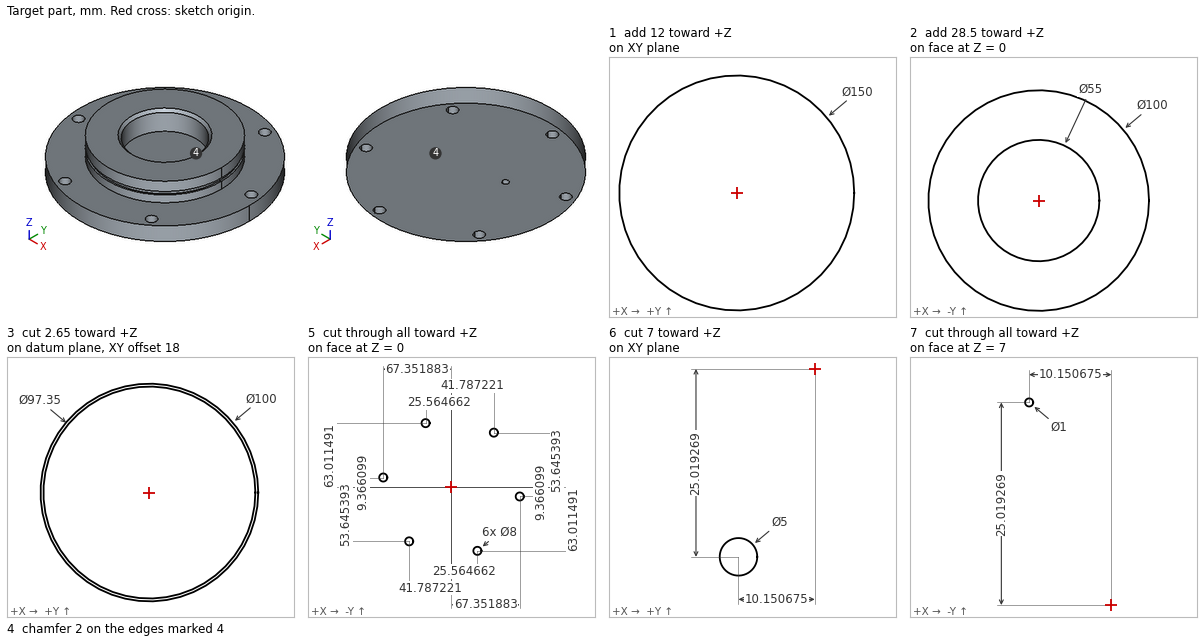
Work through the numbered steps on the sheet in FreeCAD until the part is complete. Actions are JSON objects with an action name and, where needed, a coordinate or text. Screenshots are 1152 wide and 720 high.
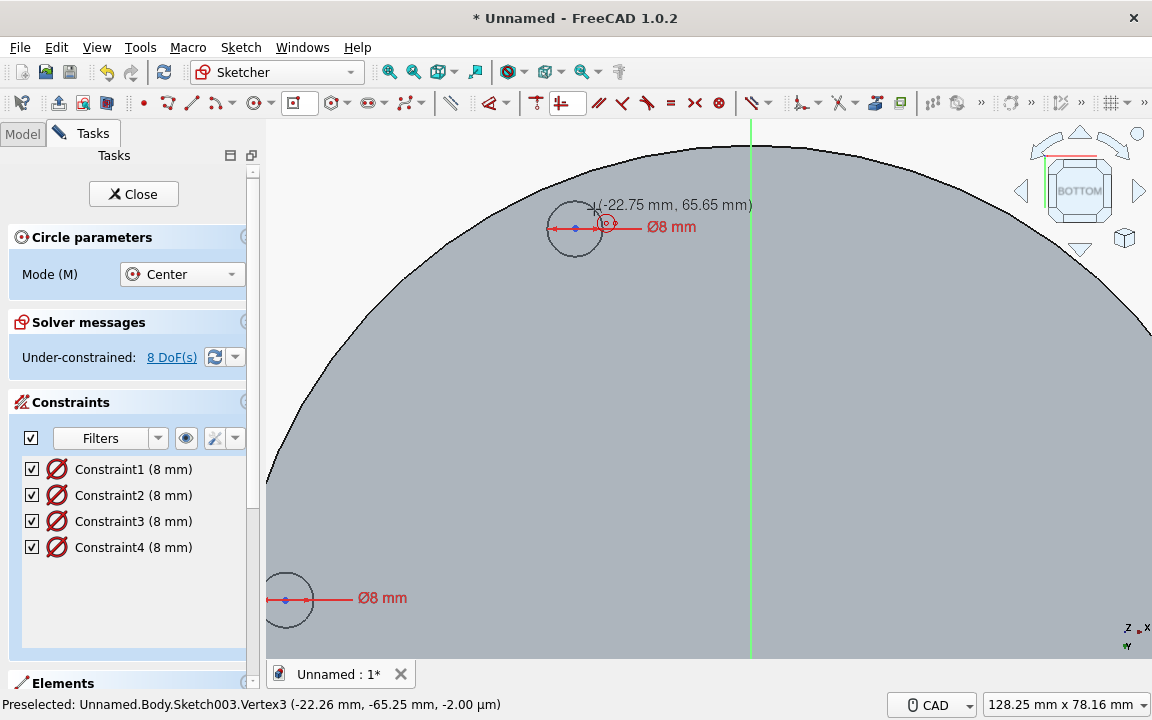
{"action": "scroll", "coordinate": [576, 229], "scroll_direction": "down", "scroll_amount": 5}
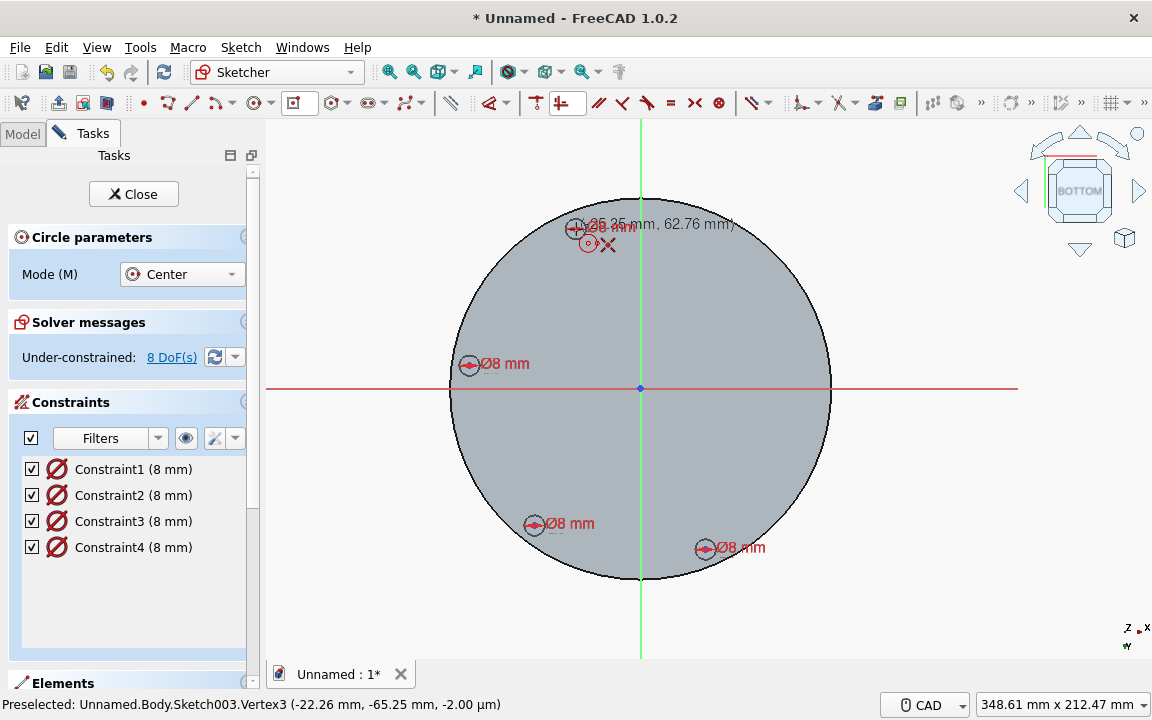
{"action": "scroll", "coordinate": [747, 253], "scroll_direction": "up", "scroll_amount": 5}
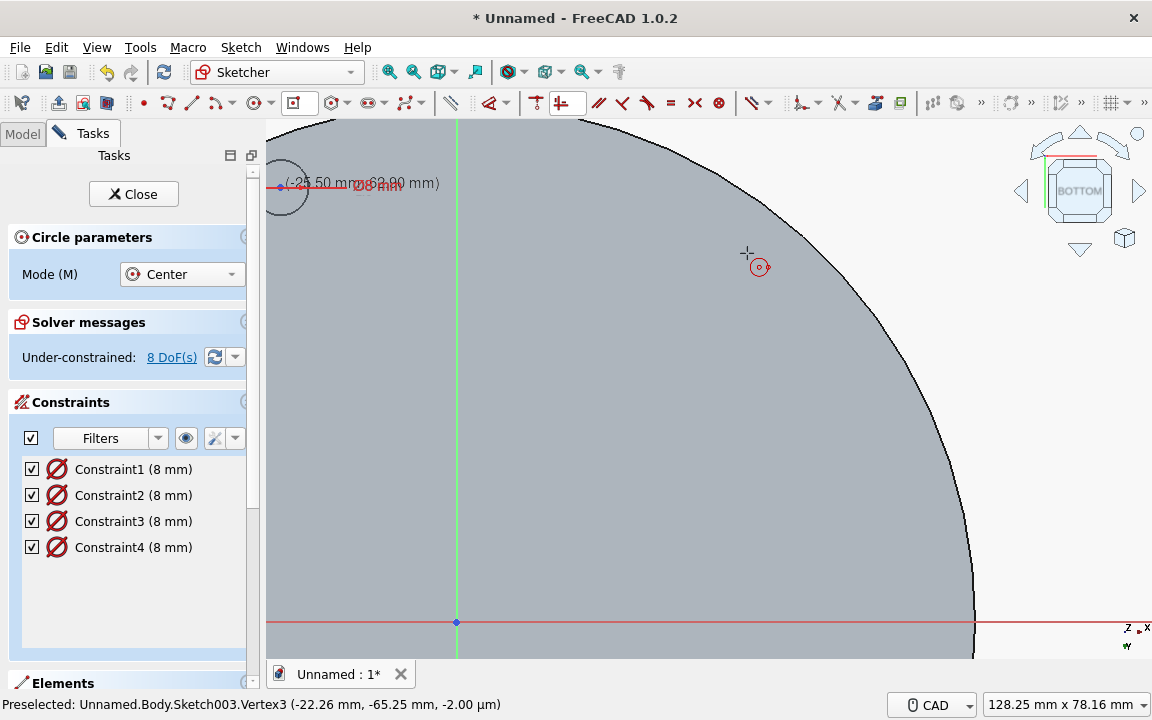
{"action": "left_click", "coordinate": [746, 252]}
{"action": "mouse_move", "coordinate": [765, 232]}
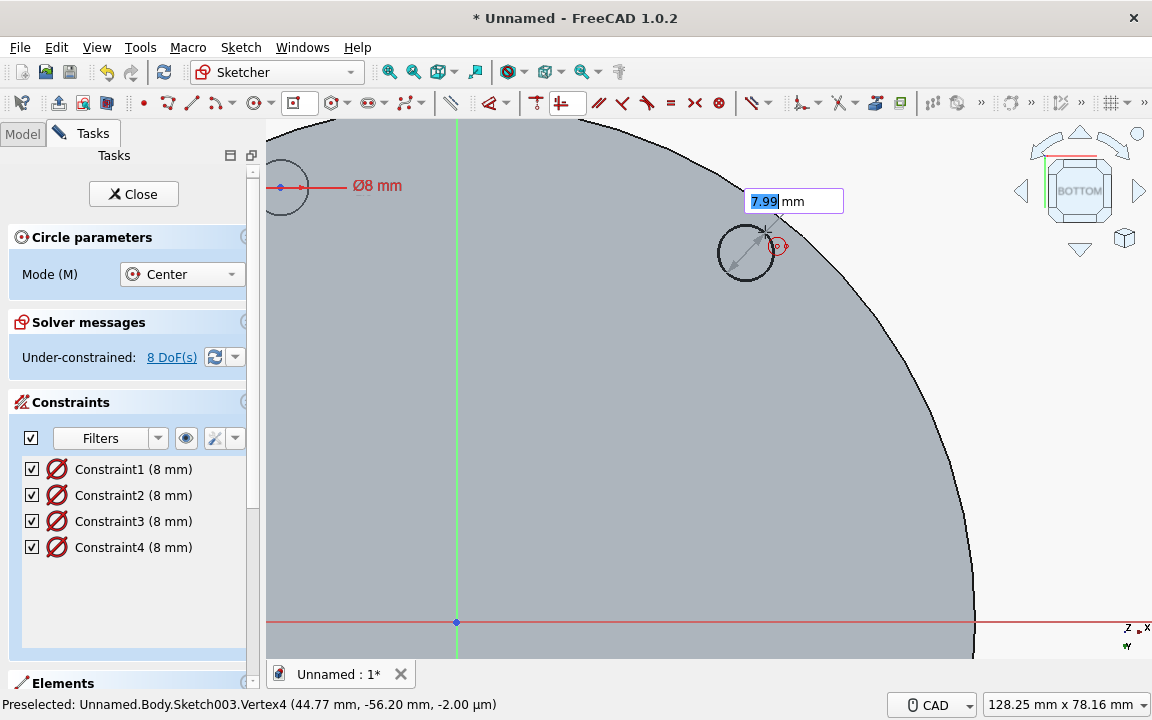
{"action": "type", "text": "8"}
{"action": "key", "text": "Return"}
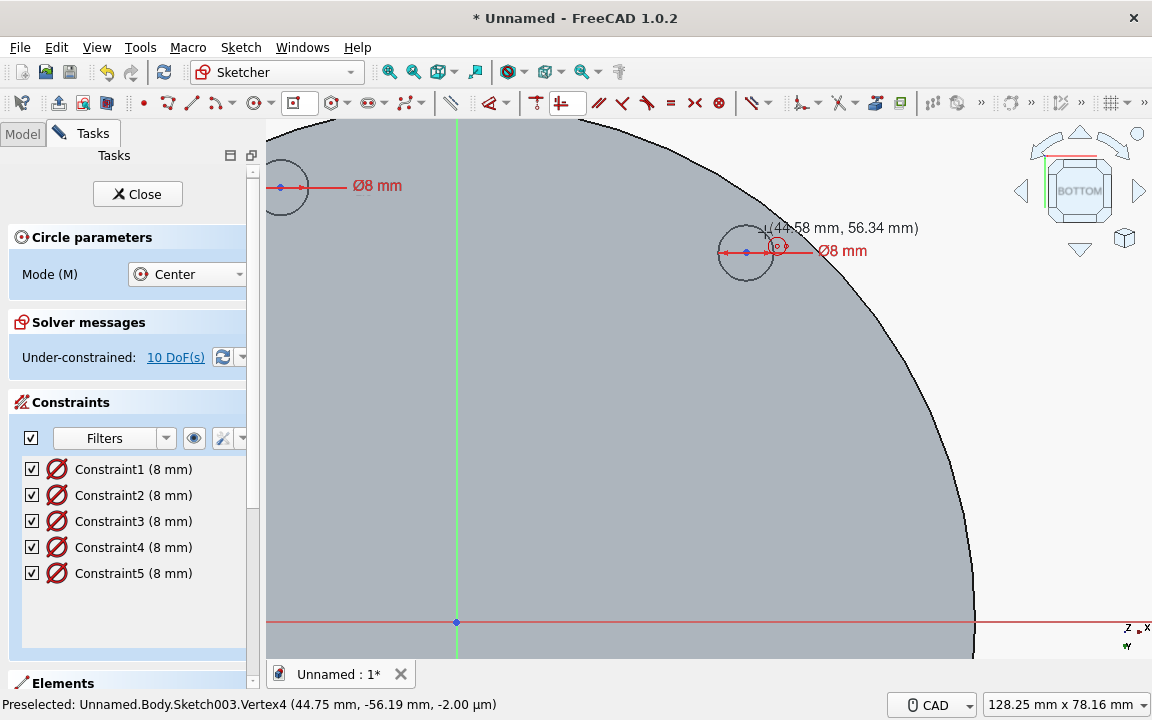
{"action": "scroll", "coordinate": [747, 253], "scroll_direction": "down", "scroll_amount": 5}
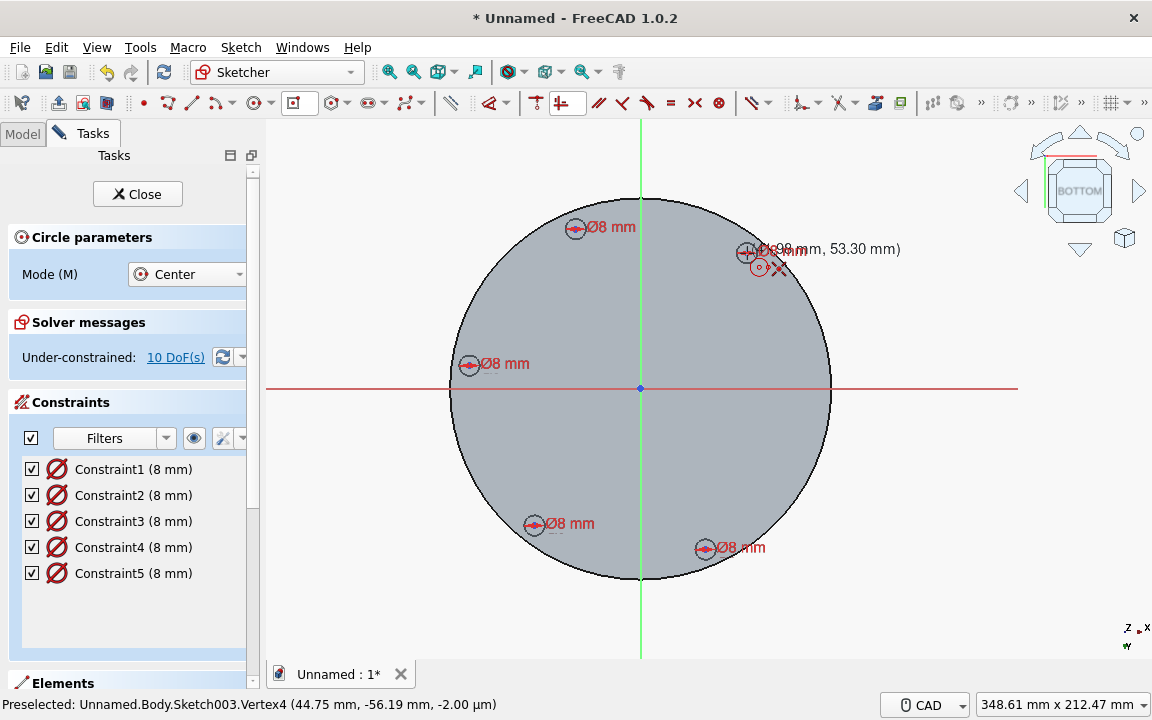
{"action": "scroll", "coordinate": [812, 413], "scroll_direction": "up", "scroll_amount": 5}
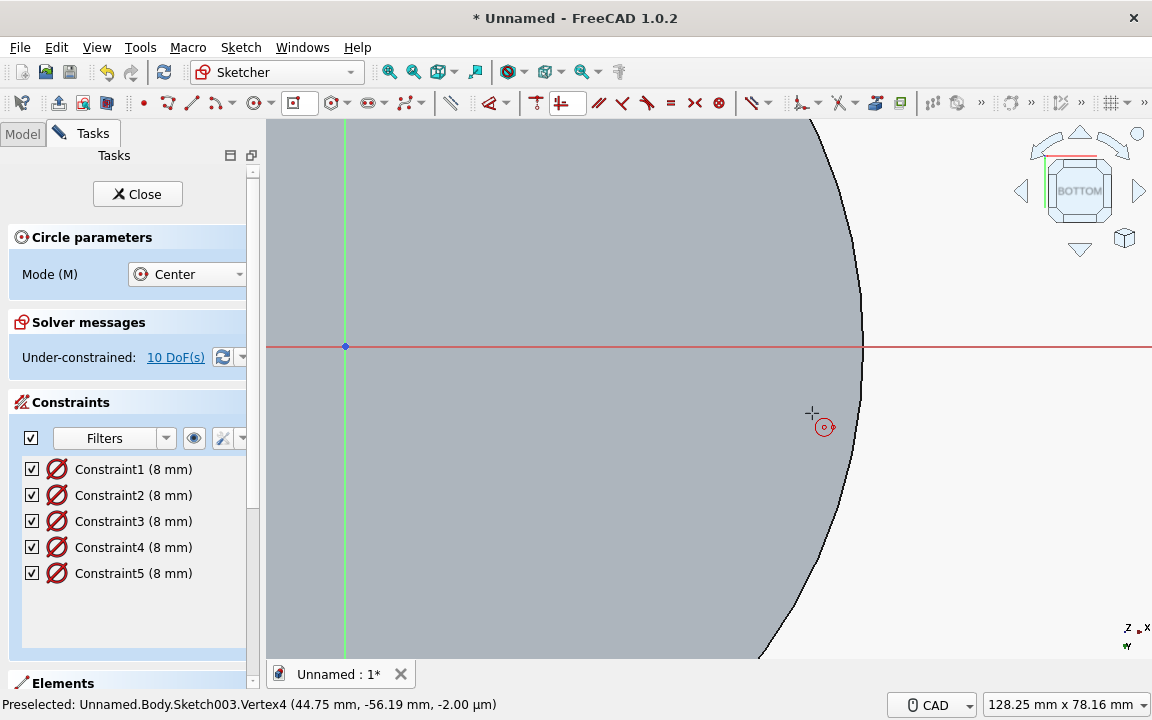
{"action": "left_click", "coordinate": [810, 412]}
{"action": "mouse_move", "coordinate": [830, 392]}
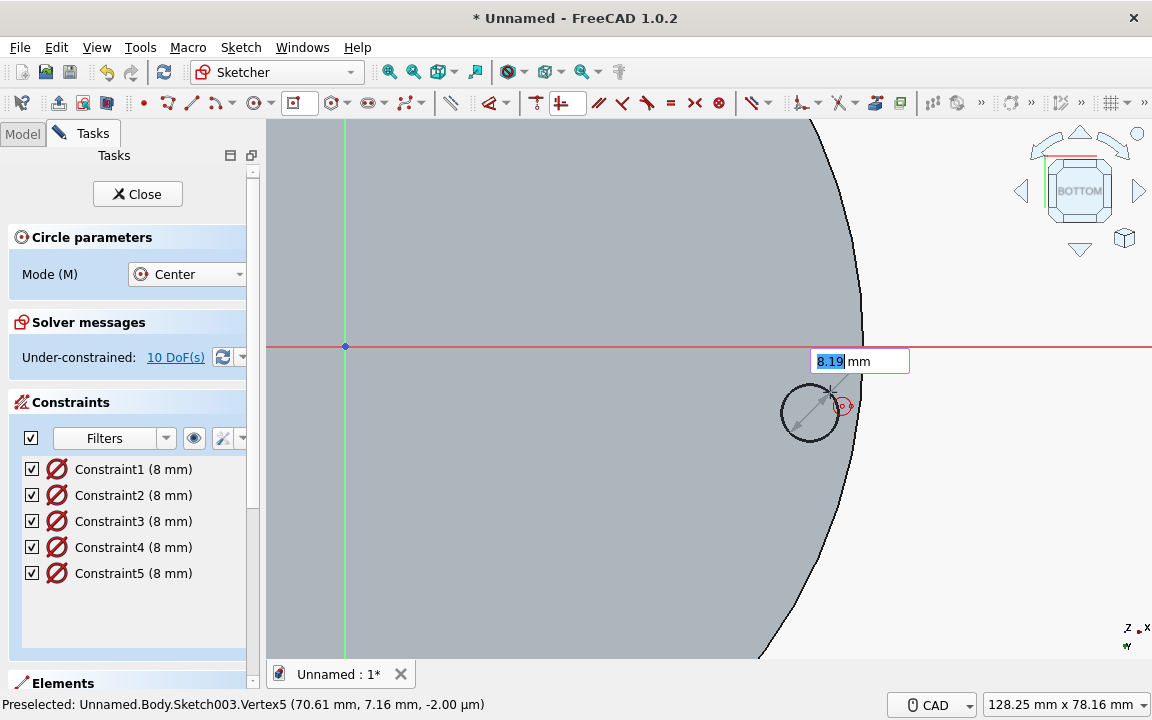
{"action": "type", "text": "8"}
{"action": "key", "text": "Return"}
{"action": "key", "text": "Escape"}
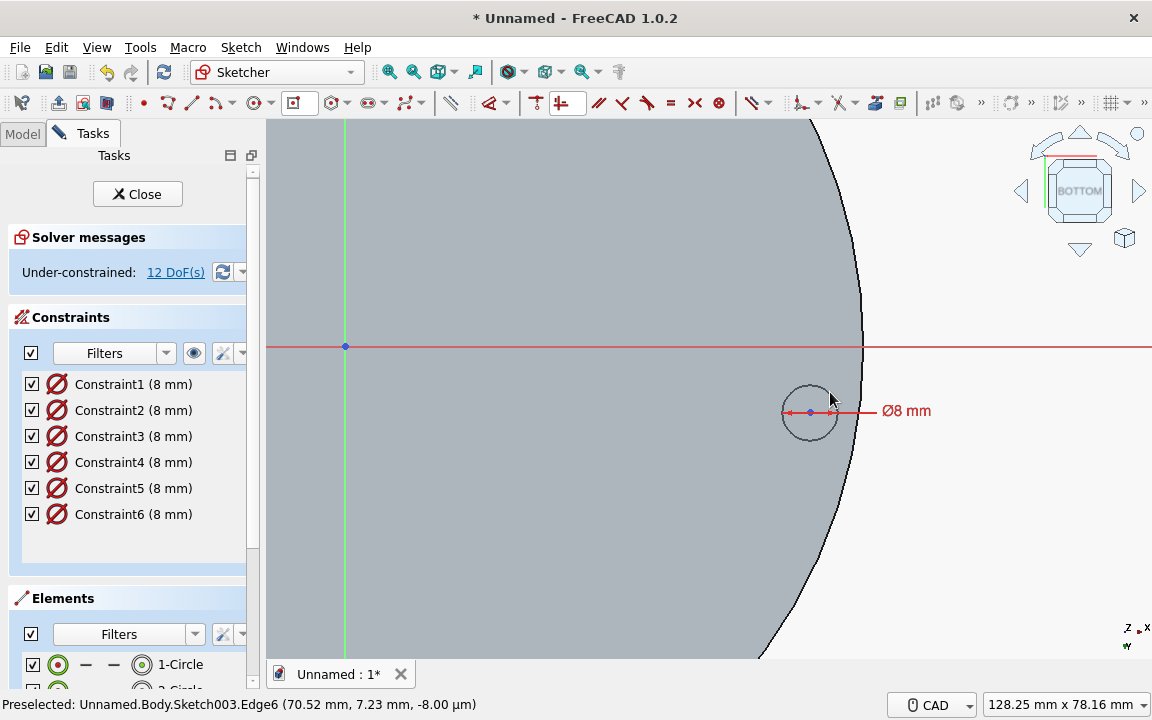
{"action": "scroll", "coordinate": [812, 414], "scroll_direction": "down", "scroll_amount": 5}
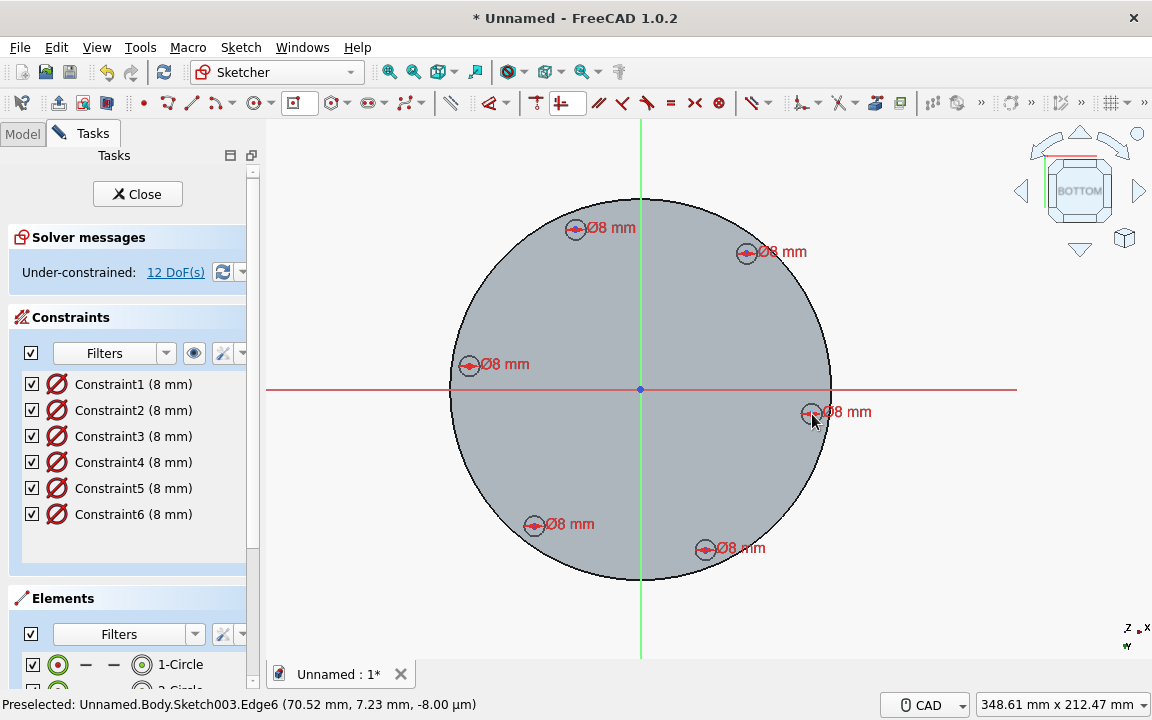
{"action": "scroll", "coordinate": [470, 366], "scroll_direction": "up", "scroll_amount": 3}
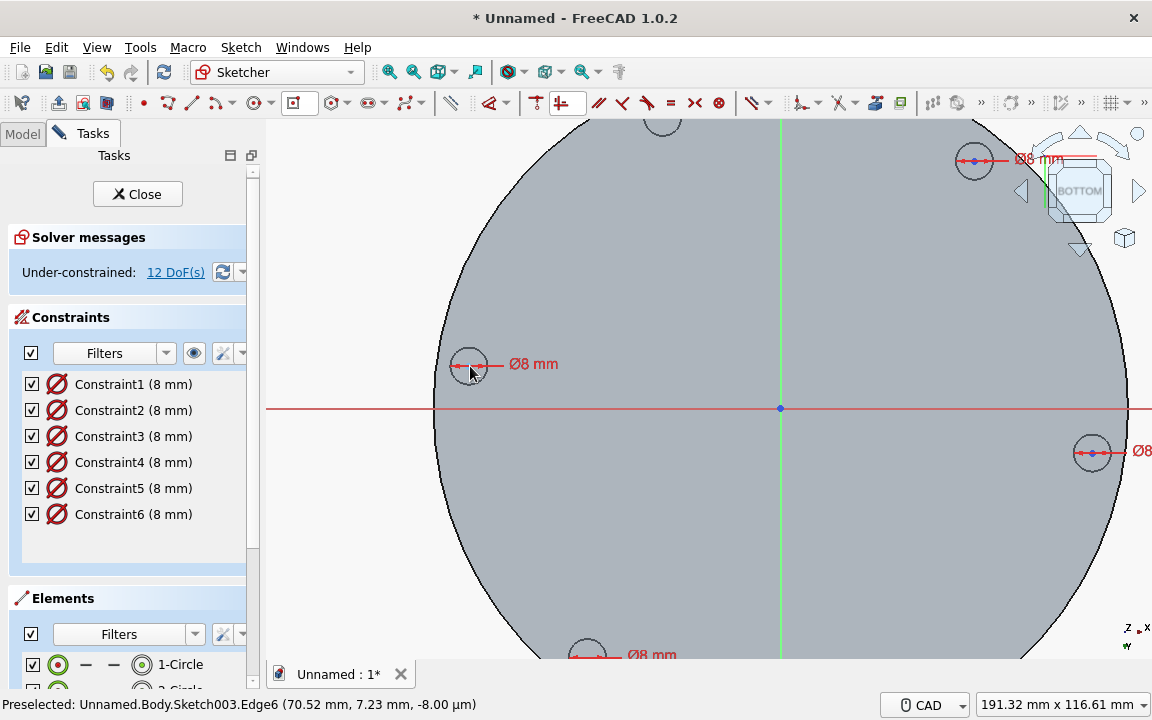
{"action": "left_click", "coordinate": [469, 366]}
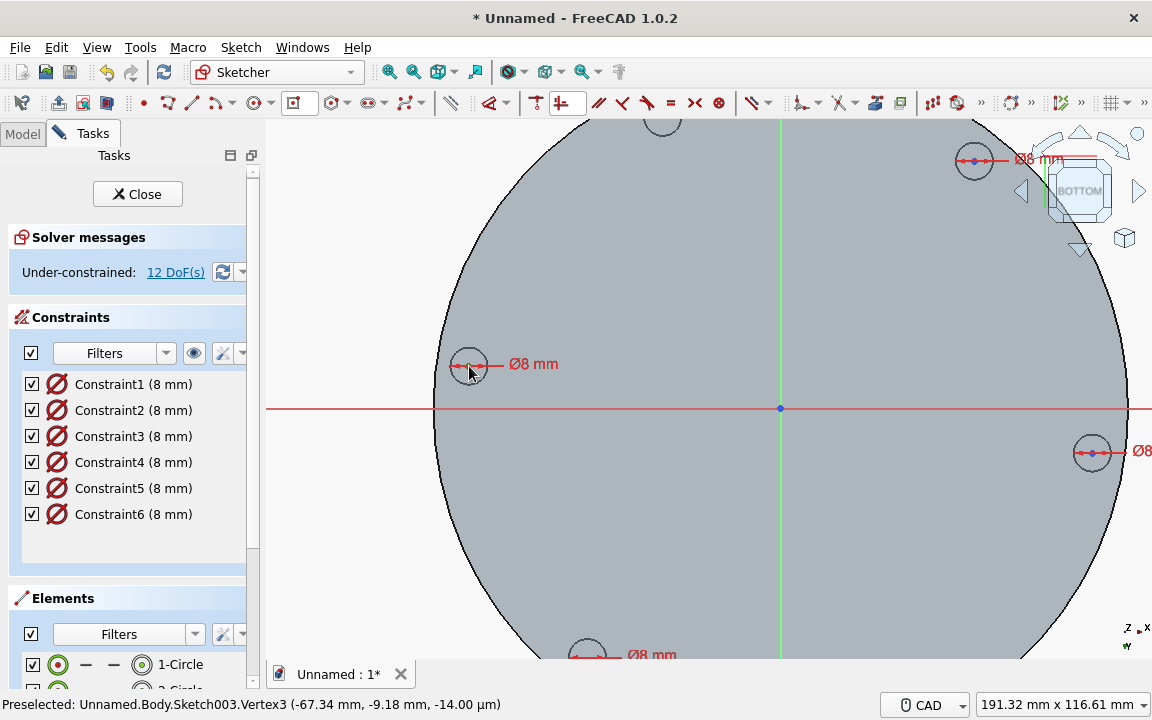
{"action": "key", "text": "i"}